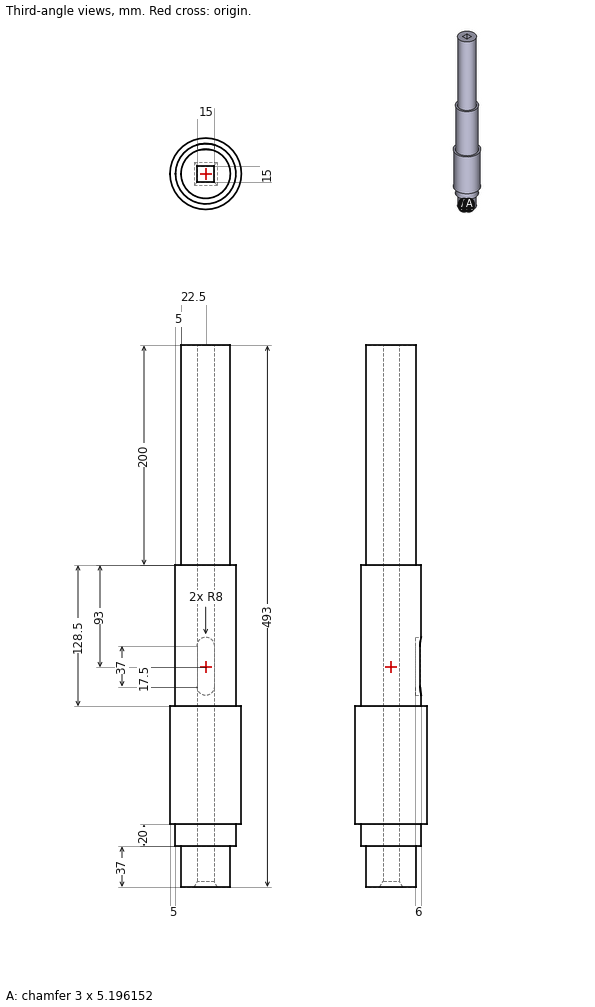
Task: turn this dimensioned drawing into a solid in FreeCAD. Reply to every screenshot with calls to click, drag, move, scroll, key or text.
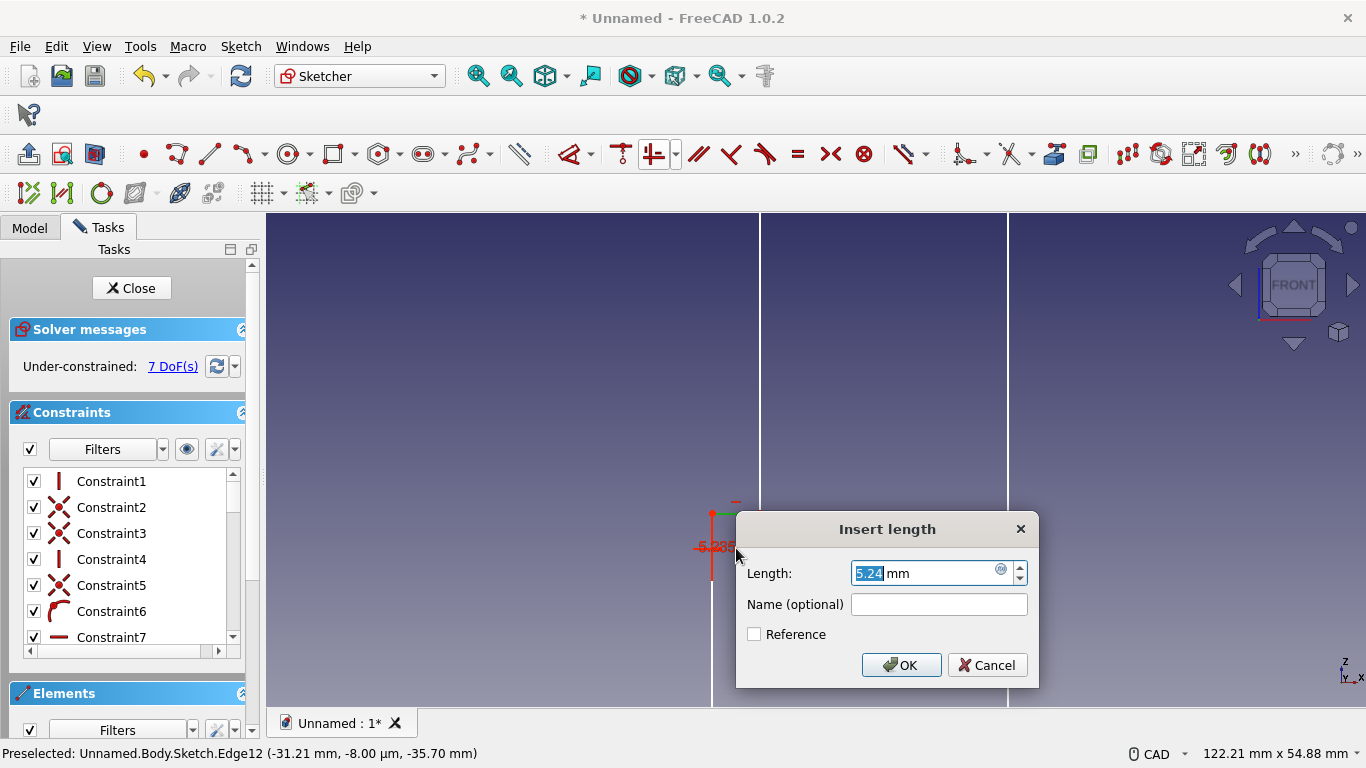
text(5)
key(Return)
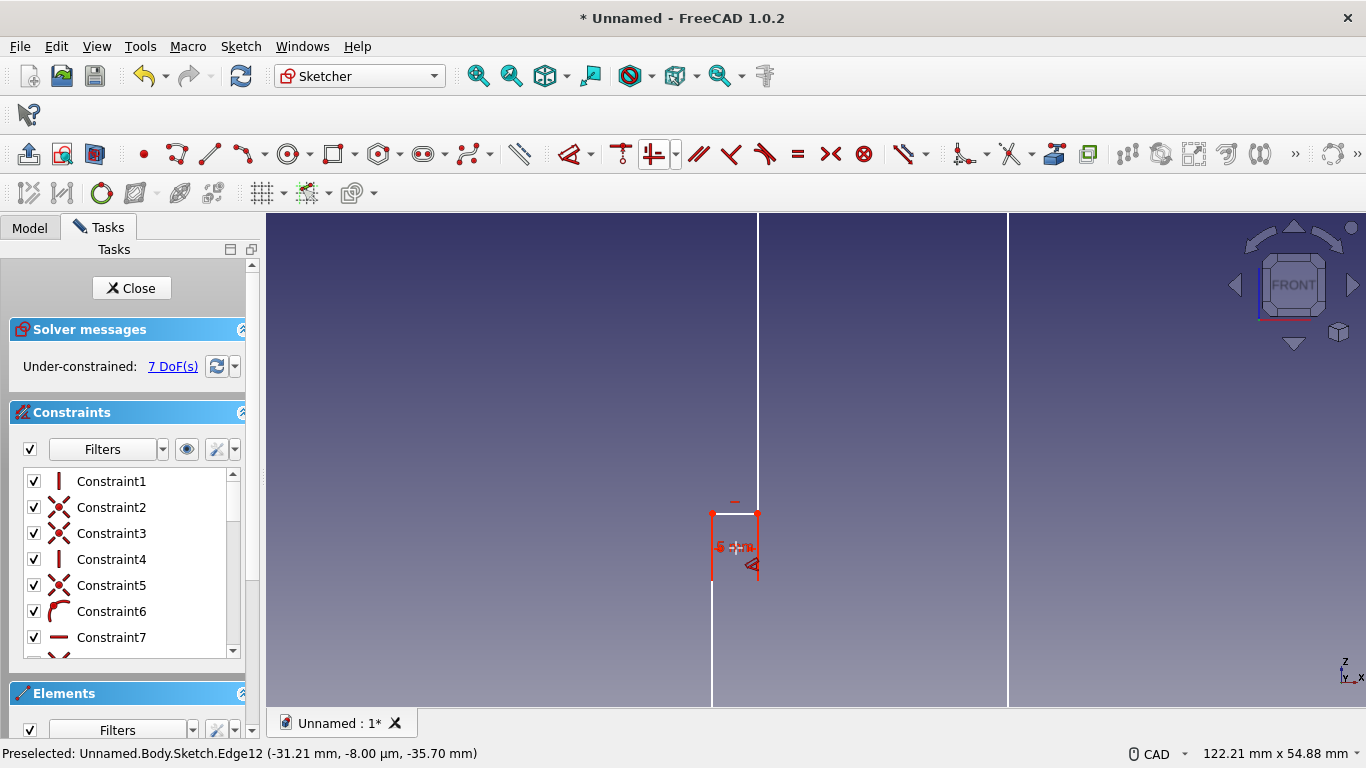
scroll(738, 515, down, 13)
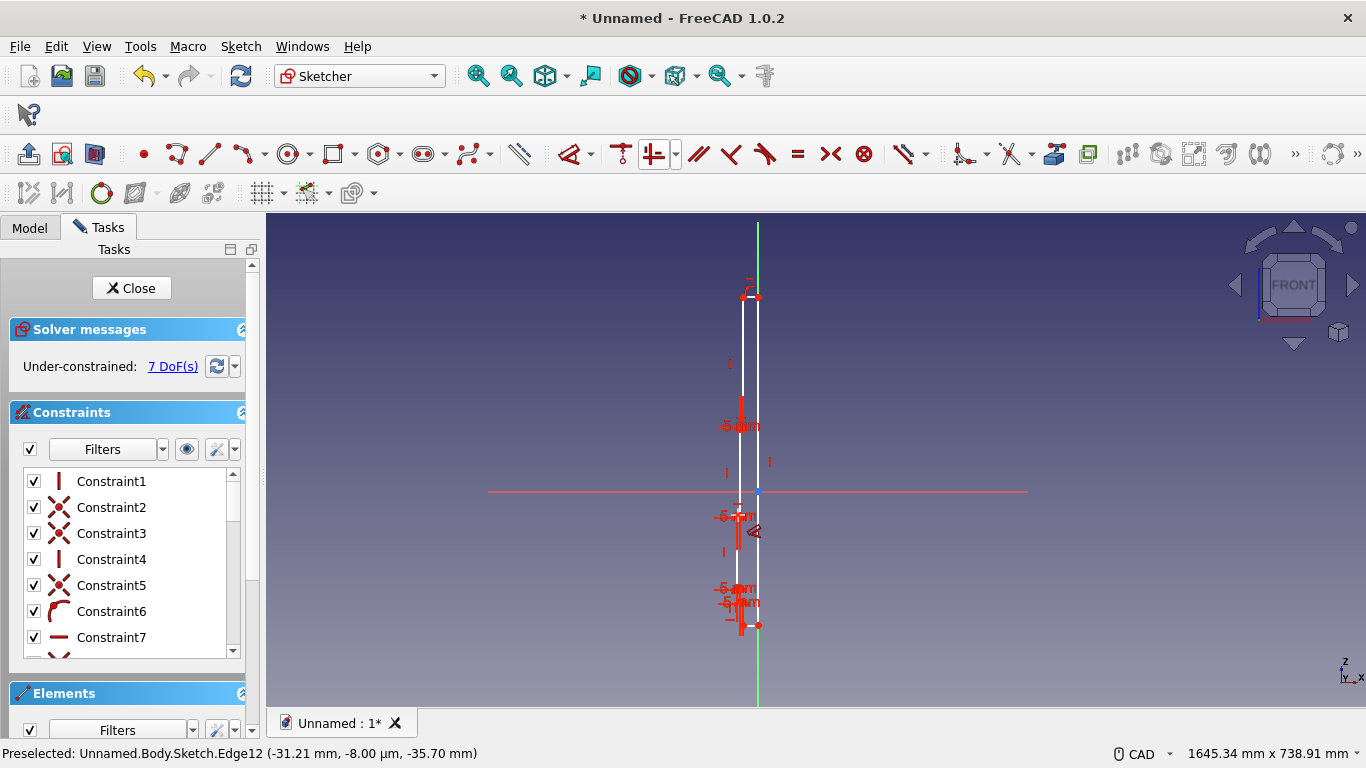
scroll(743, 619, up, 4)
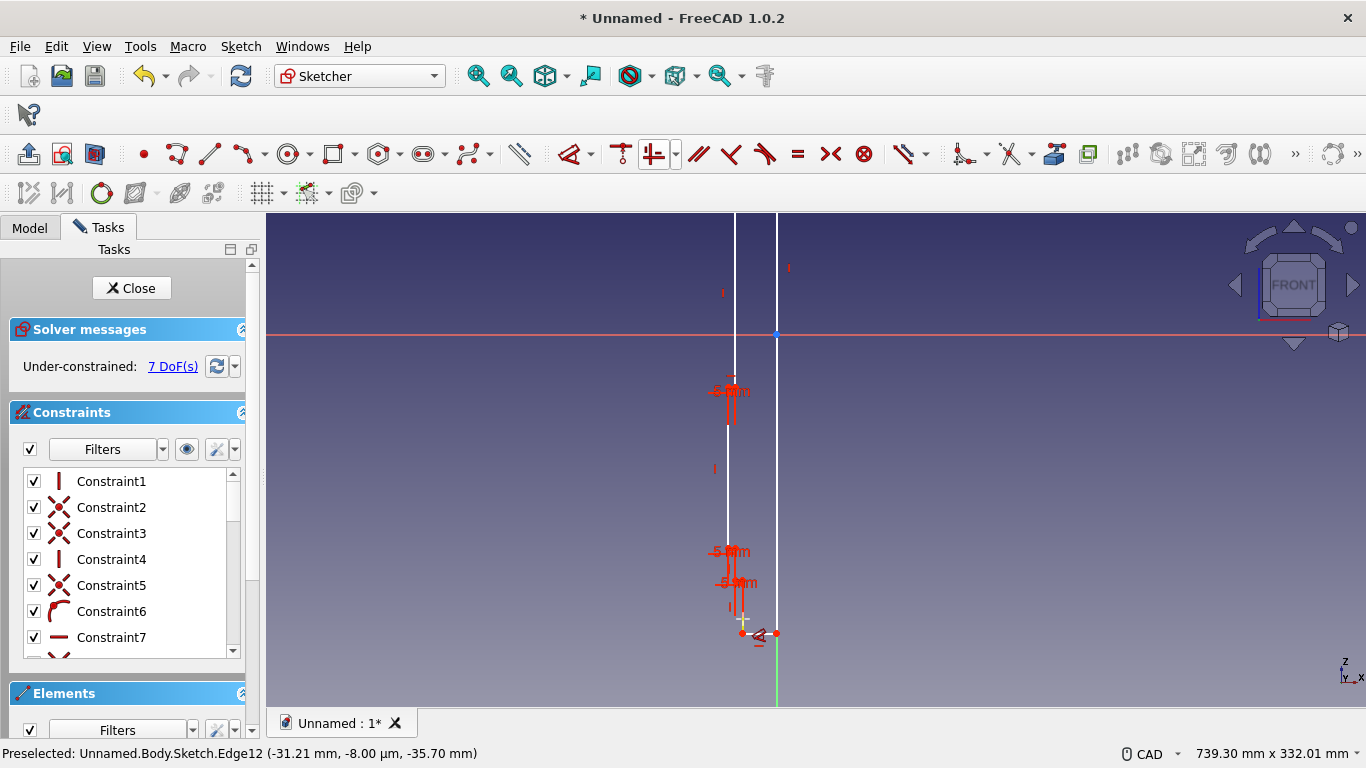
click(743, 618)
click(709, 607)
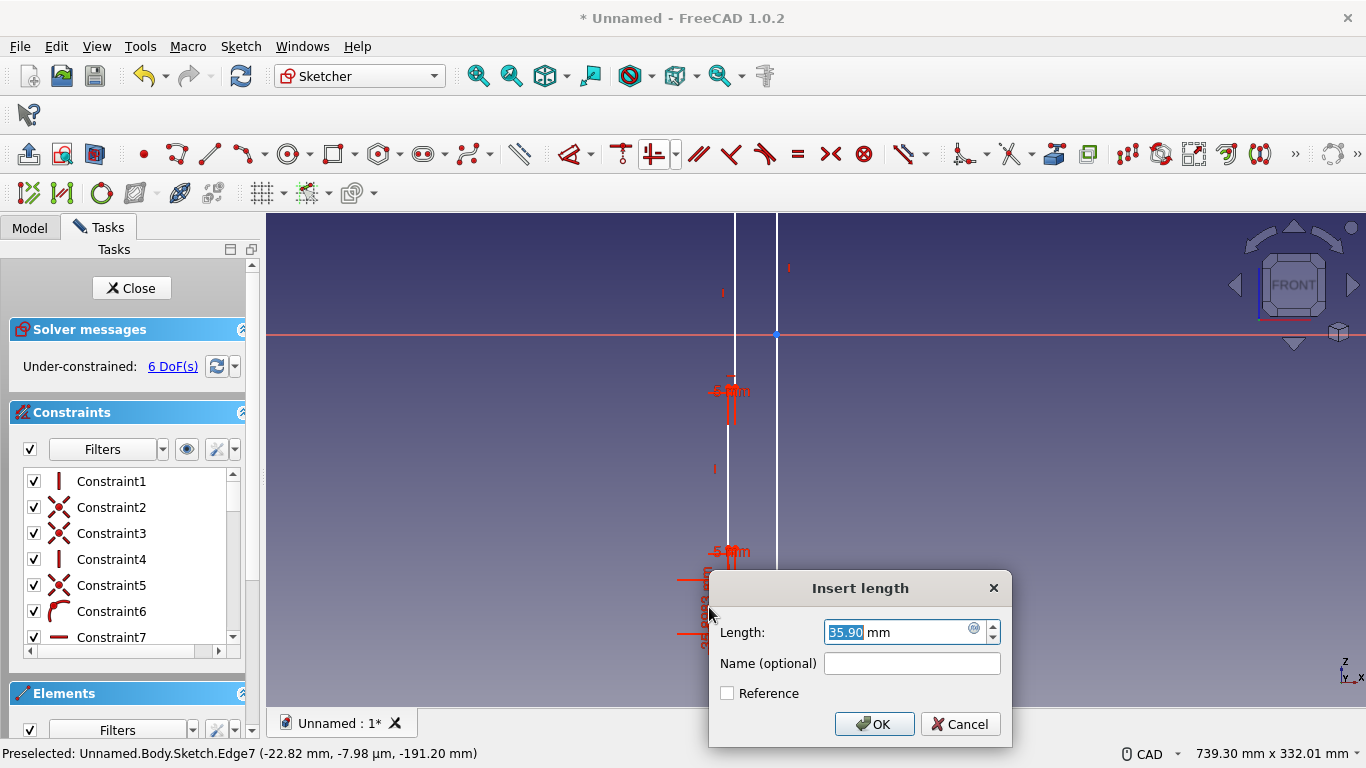
text(37)
key(Return)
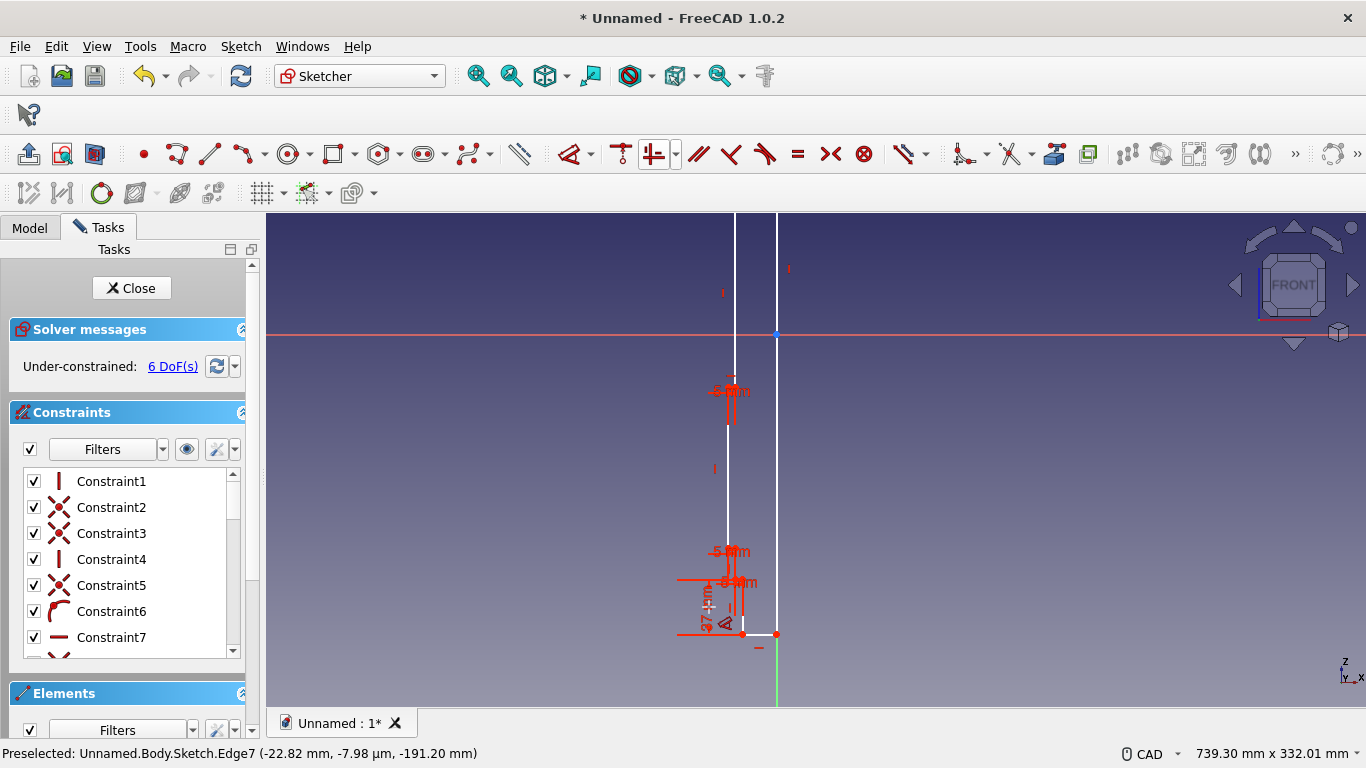
scroll(735, 571, up, 3)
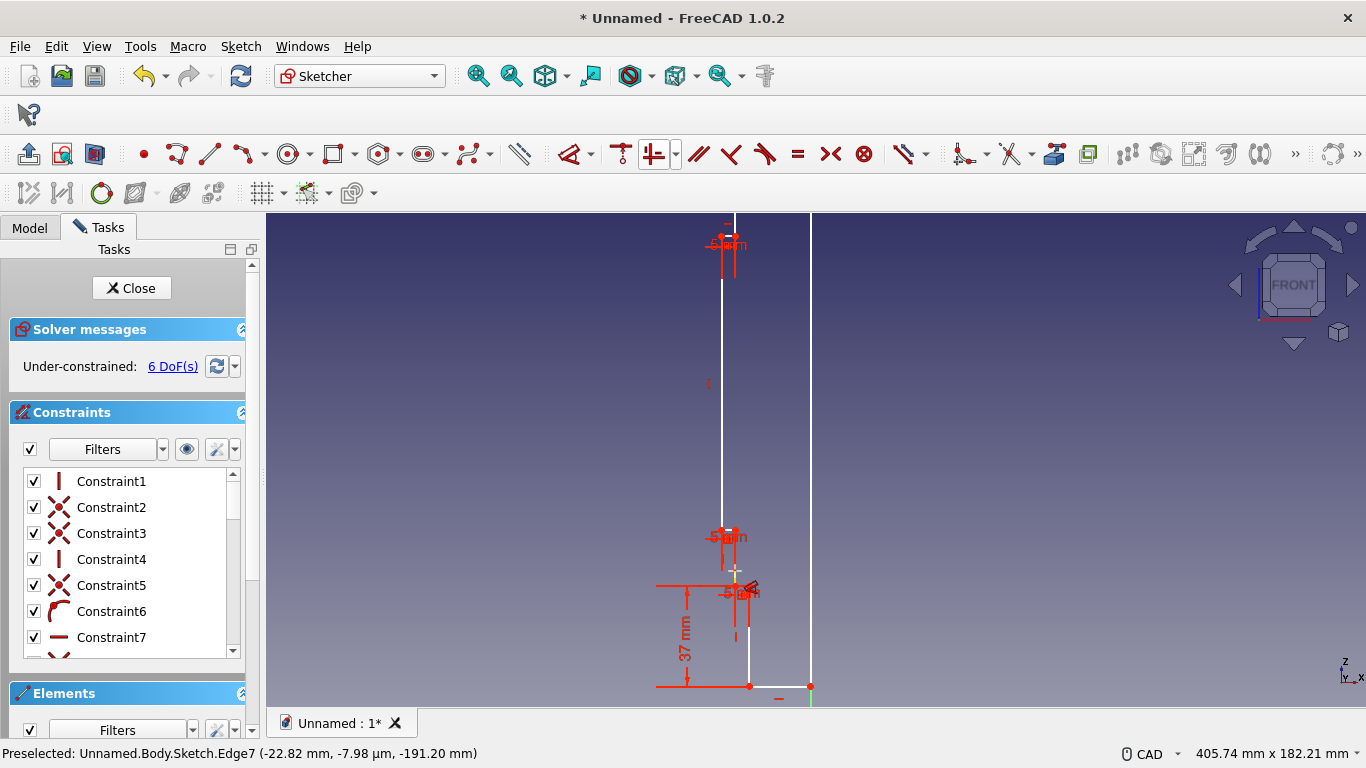
click(735, 570)
click(701, 571)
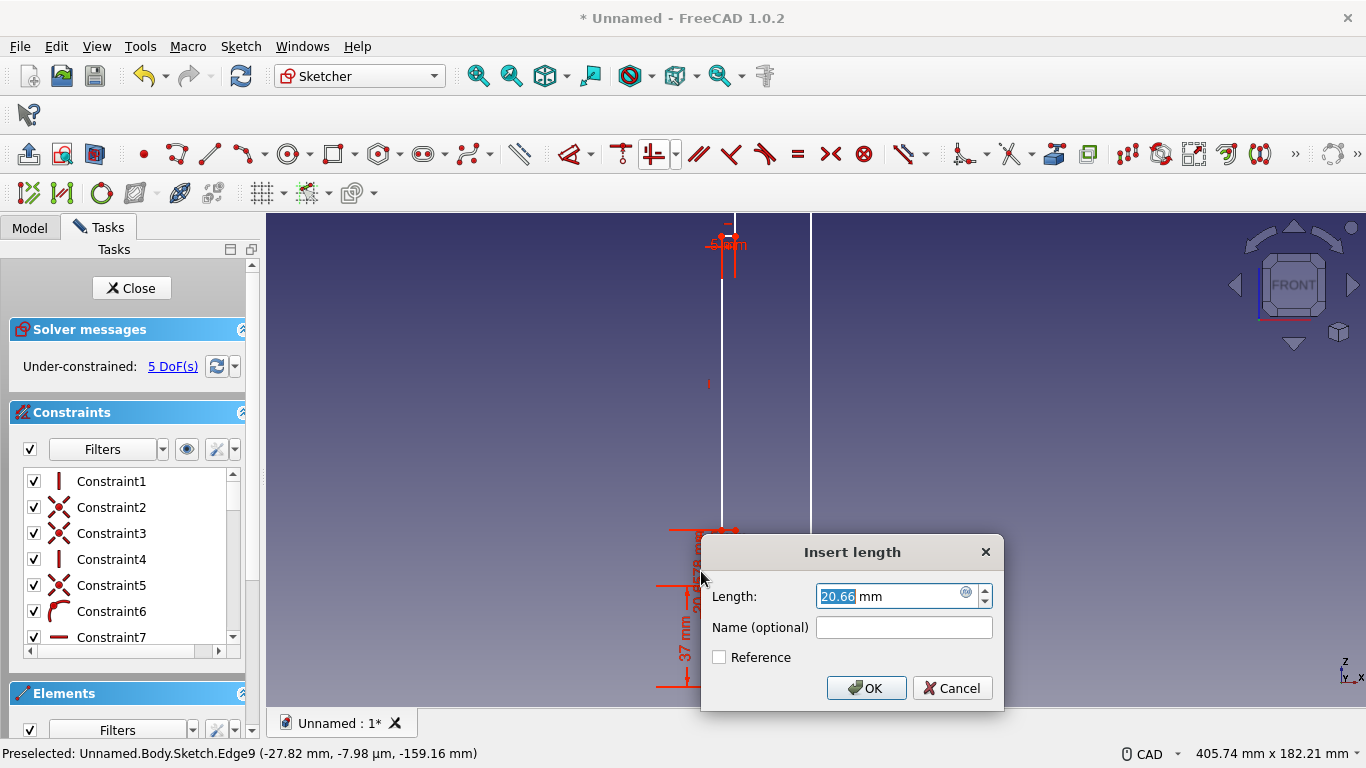
text(20)
key(Return)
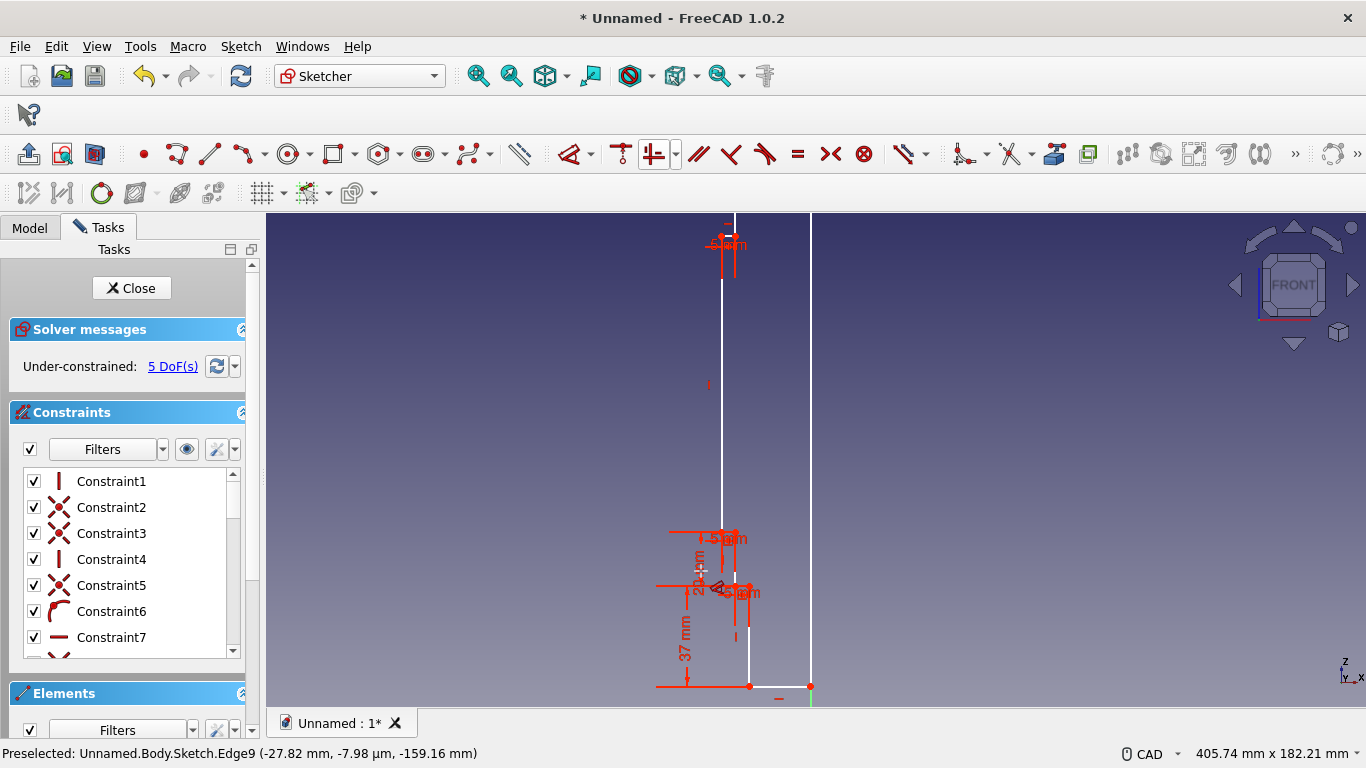
scroll(741, 606, down, 7)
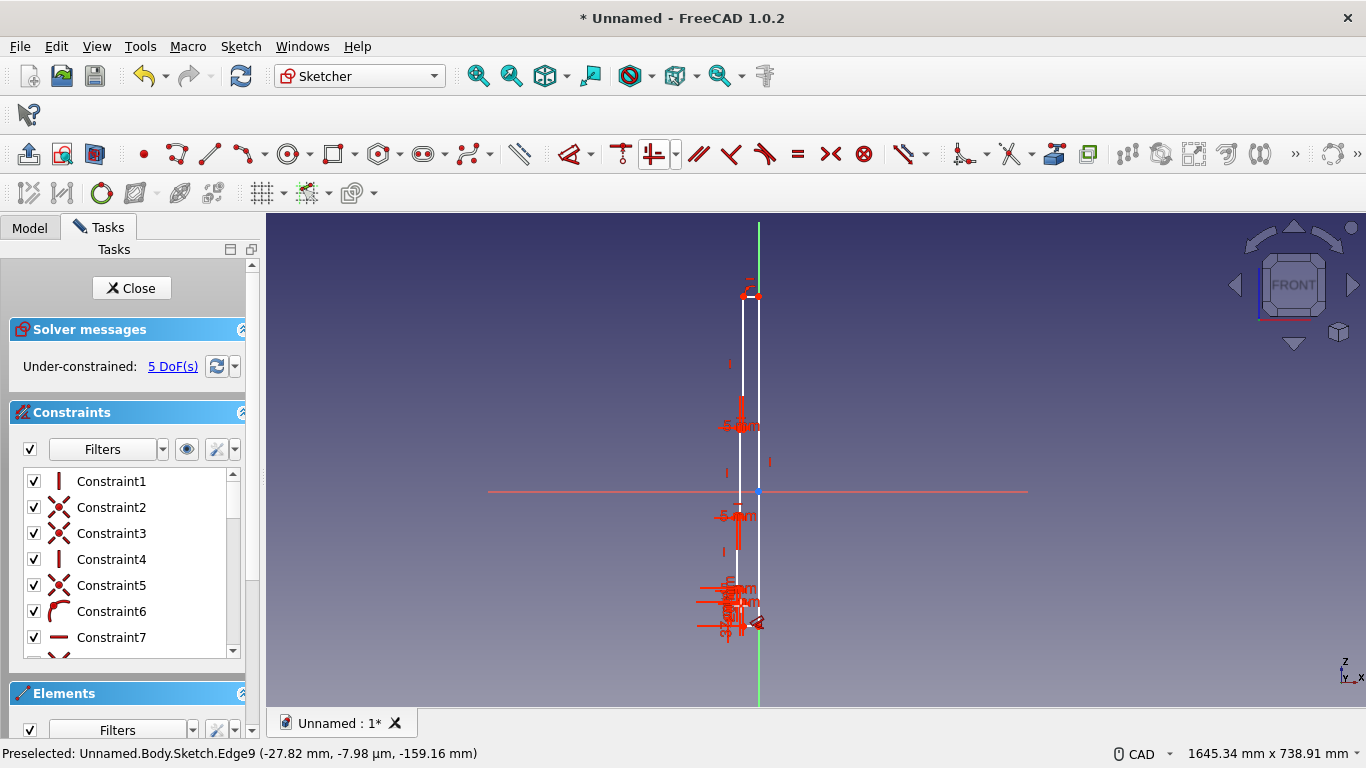
click(743, 390)
click(709, 363)